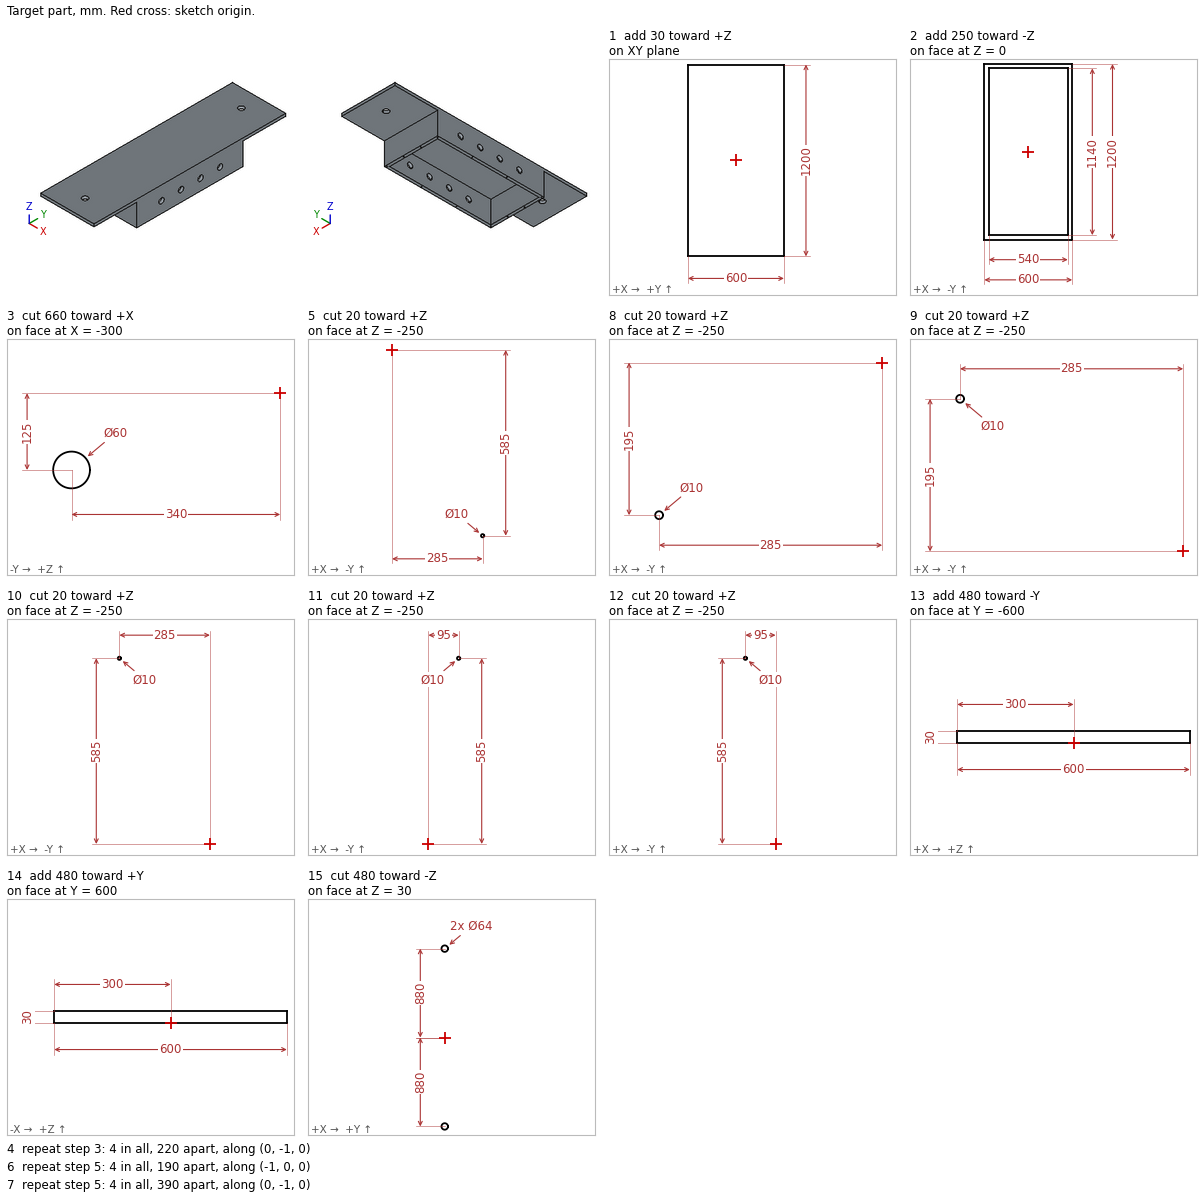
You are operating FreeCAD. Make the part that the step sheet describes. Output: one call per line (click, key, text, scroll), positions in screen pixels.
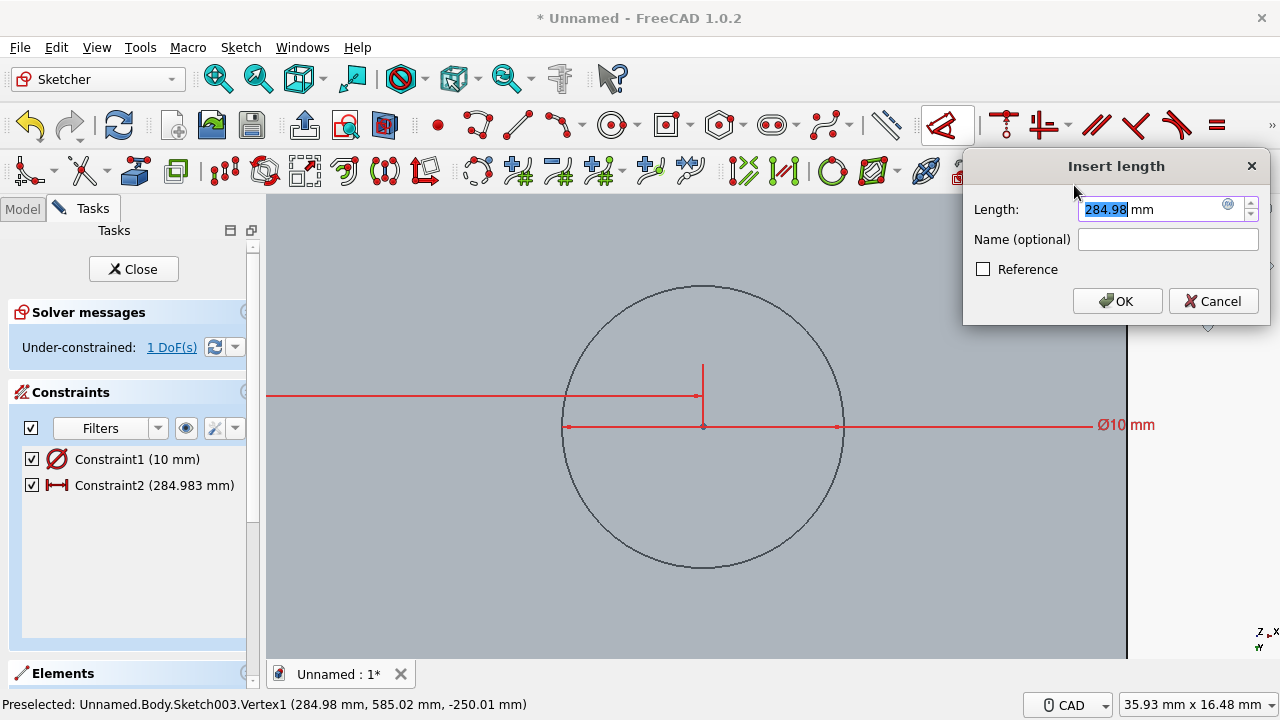
text(285)
key(Return)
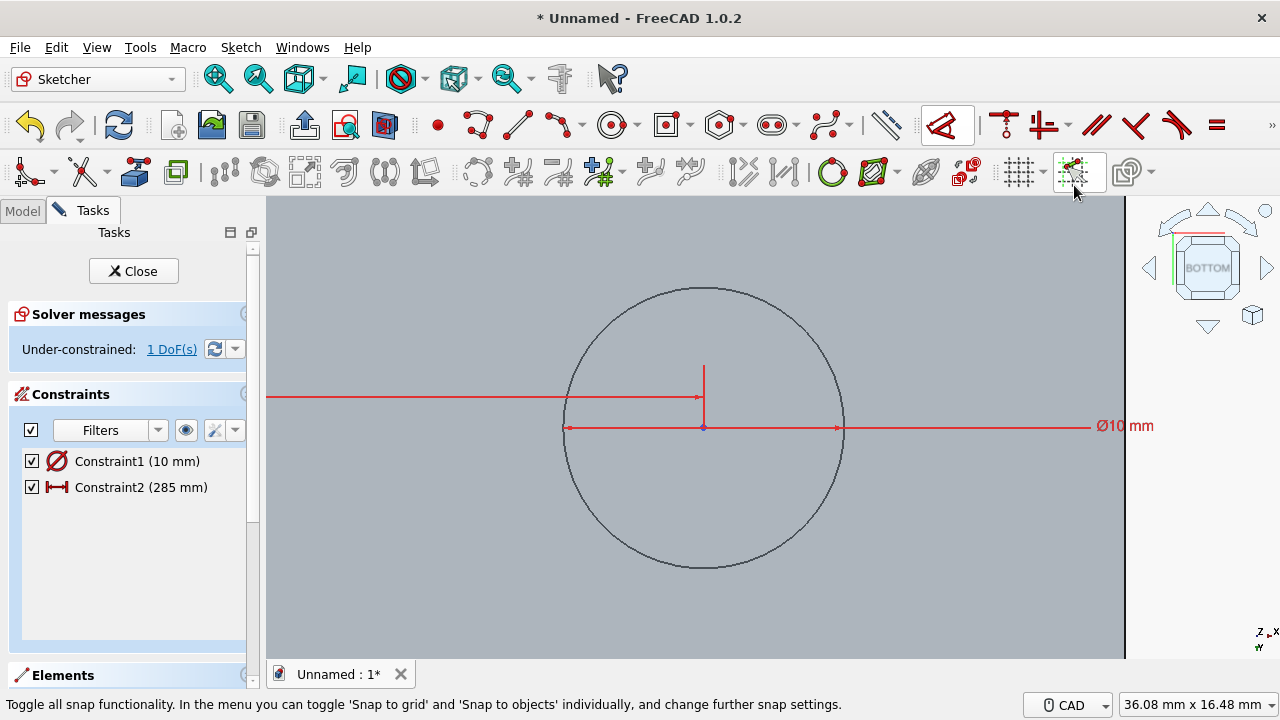
click(704, 428)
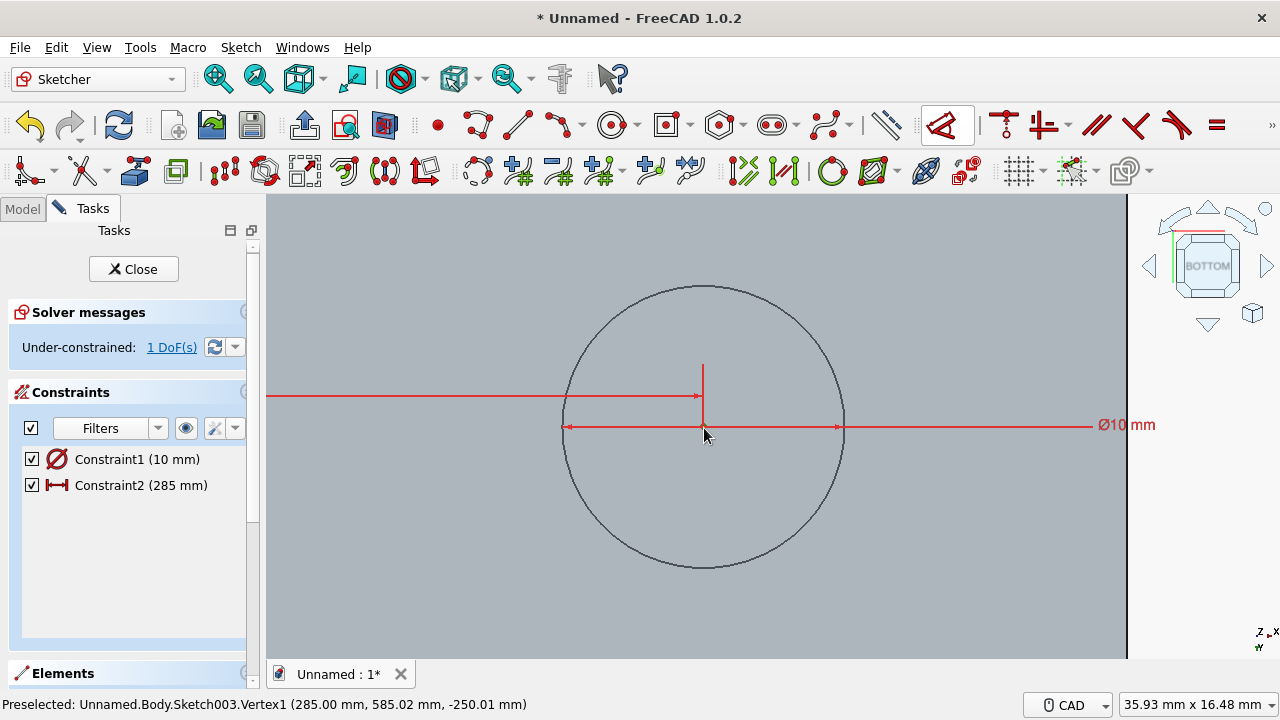
click(968, 126)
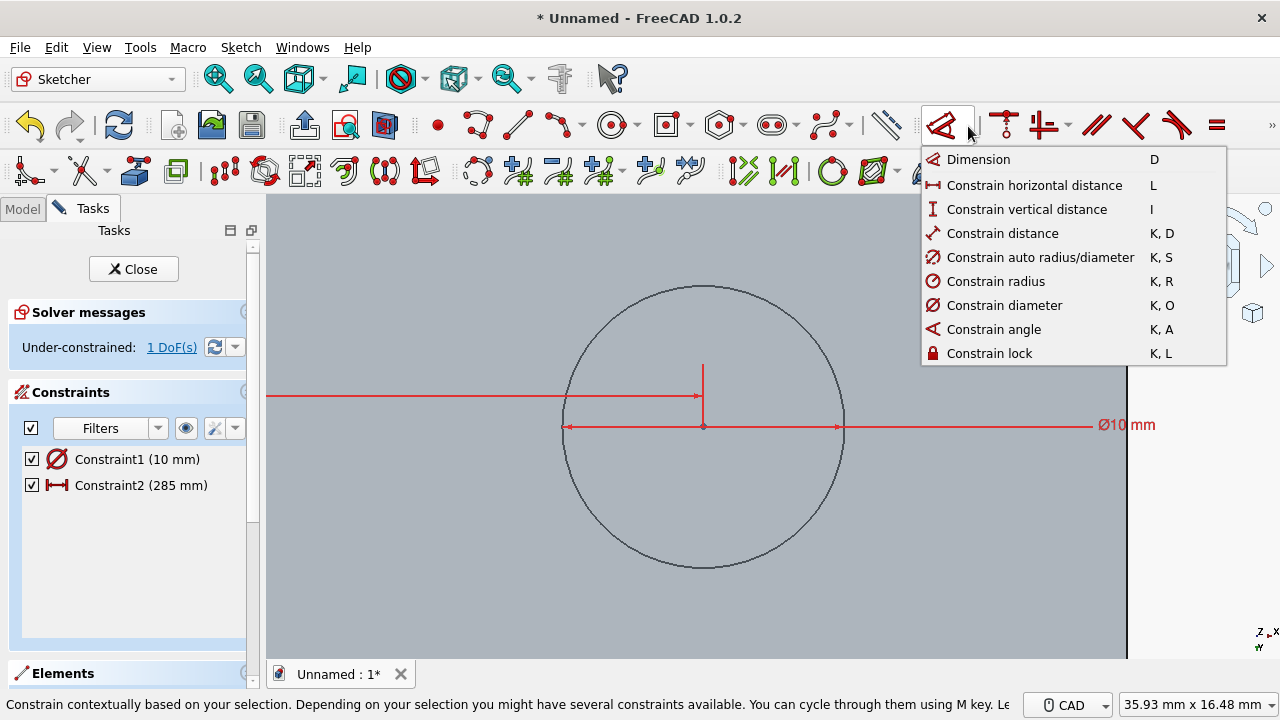
click(1074, 209)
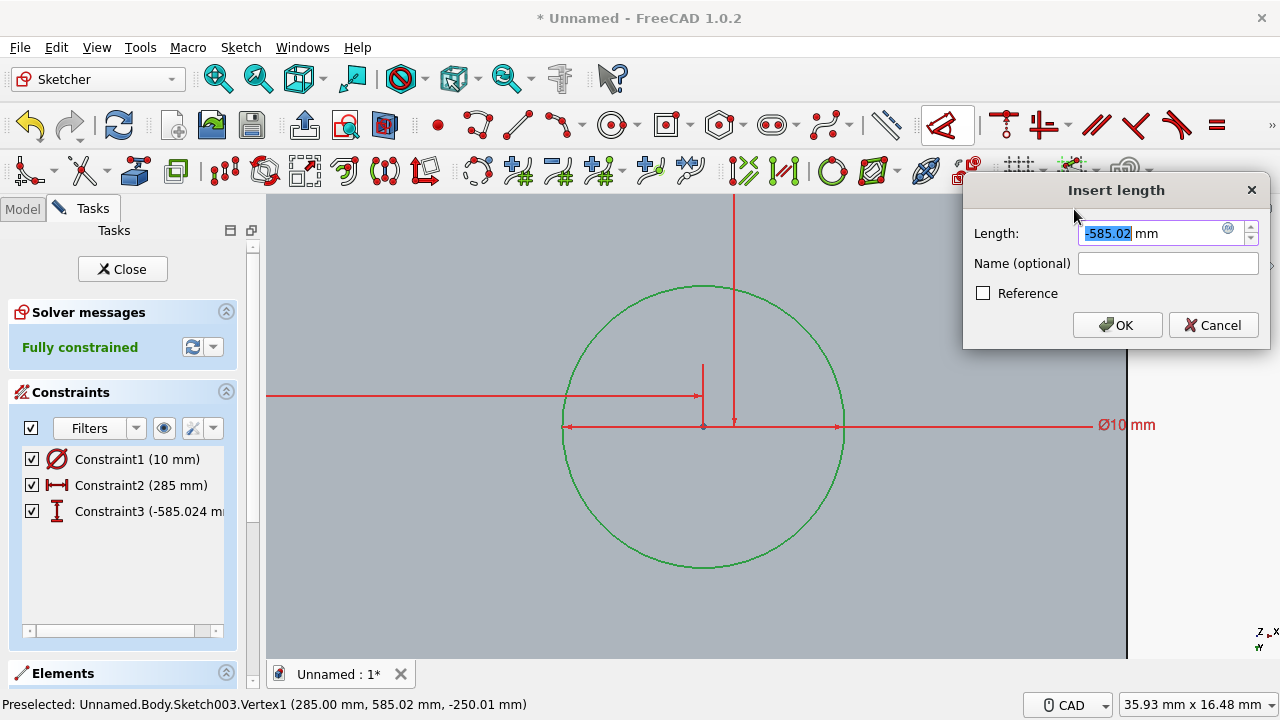
text(-585)
key(Return)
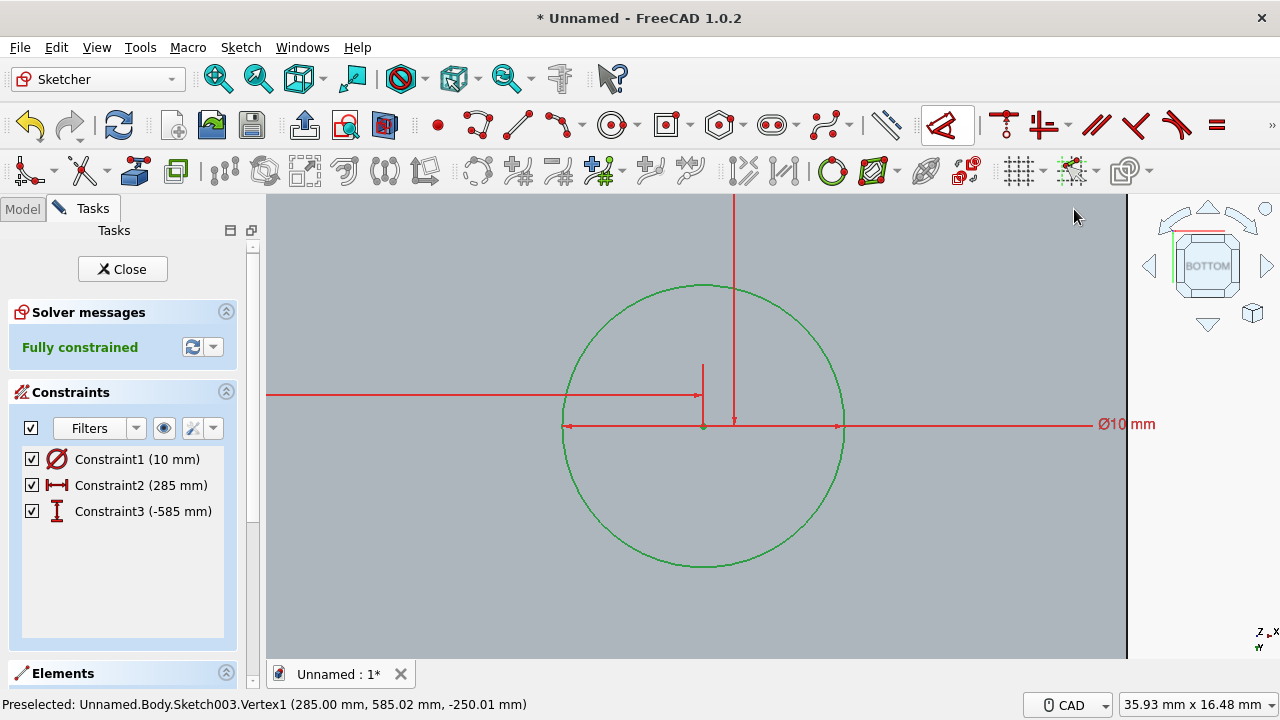
click(123, 269)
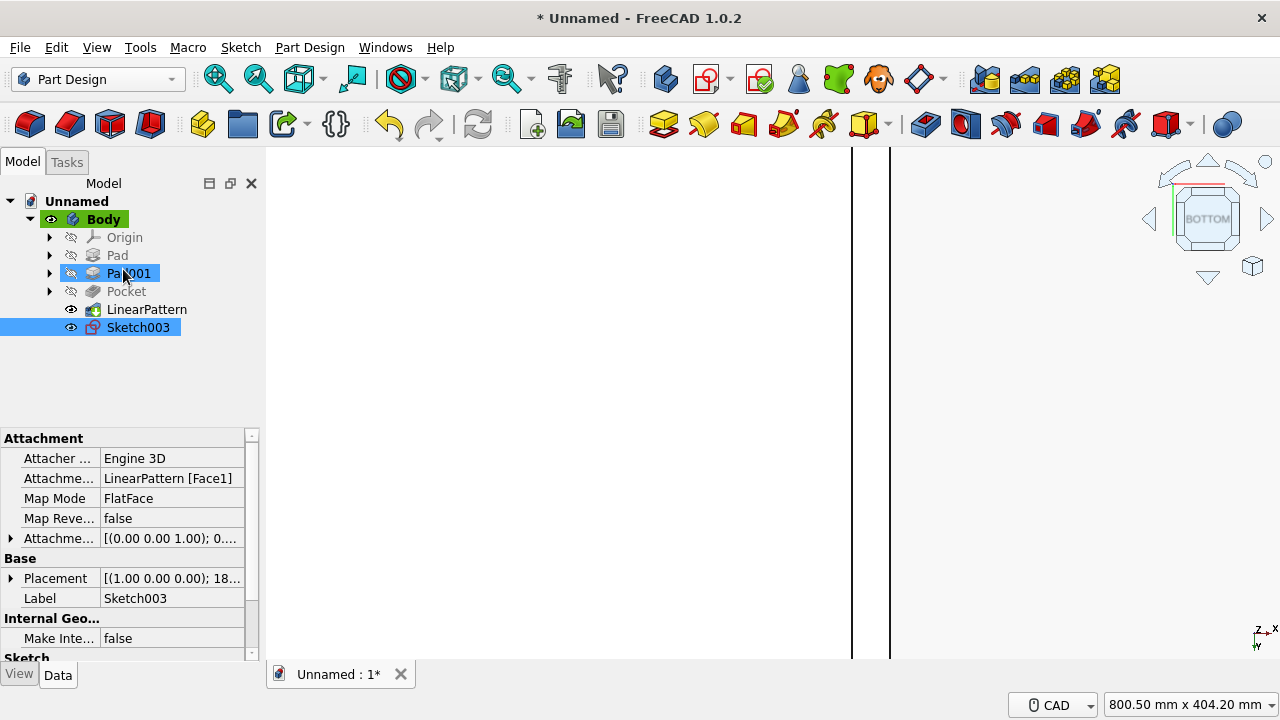
click(926, 124)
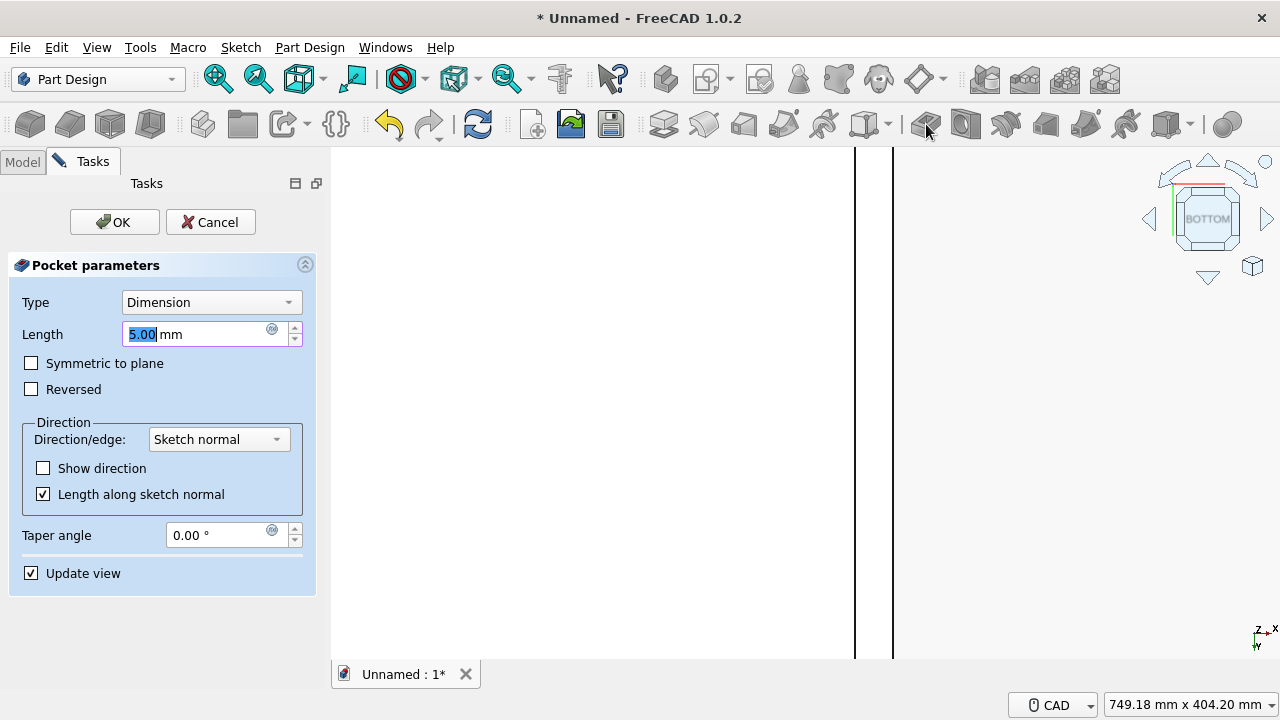
text(20)
key(Tab)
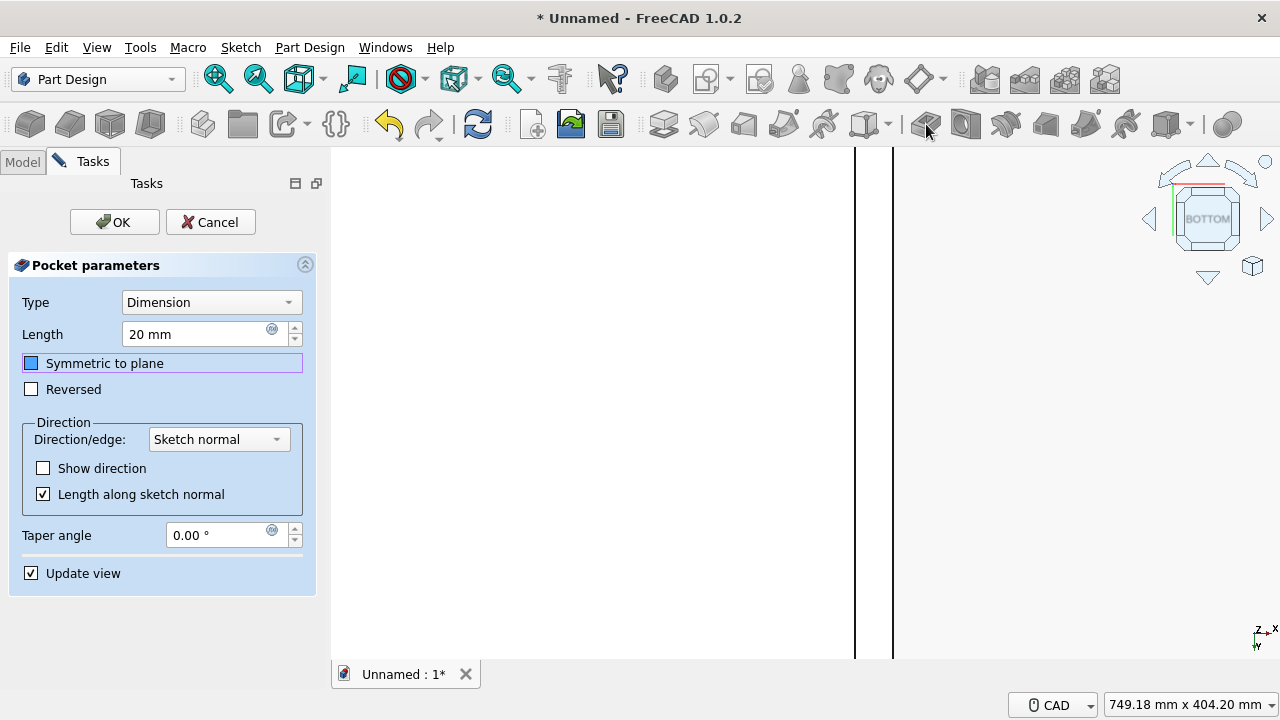
click(115, 222)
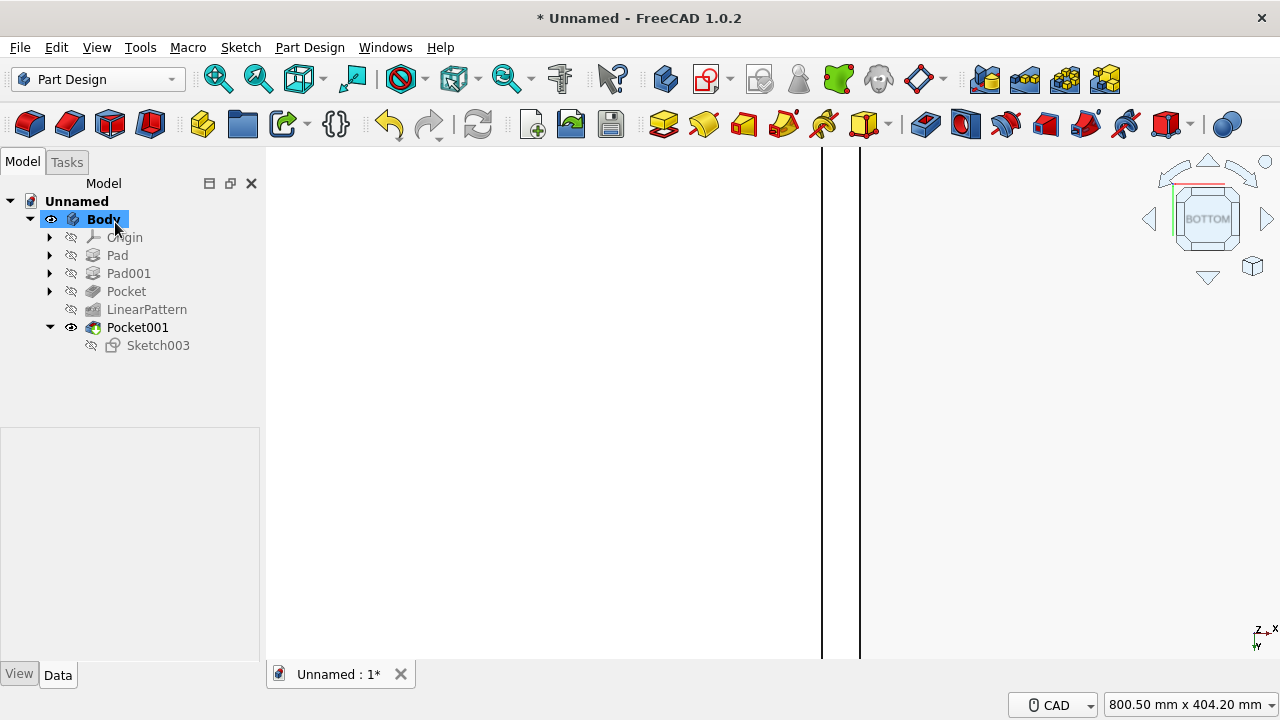
click(220, 80)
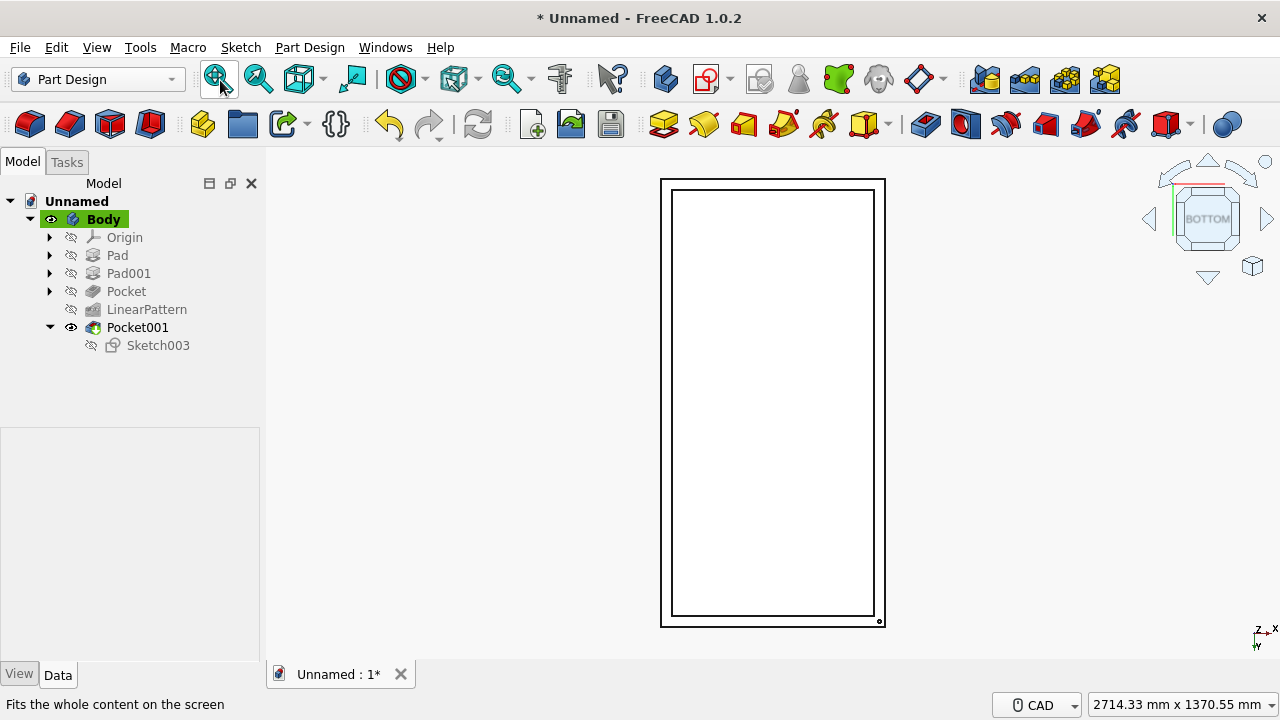
click(116, 327)